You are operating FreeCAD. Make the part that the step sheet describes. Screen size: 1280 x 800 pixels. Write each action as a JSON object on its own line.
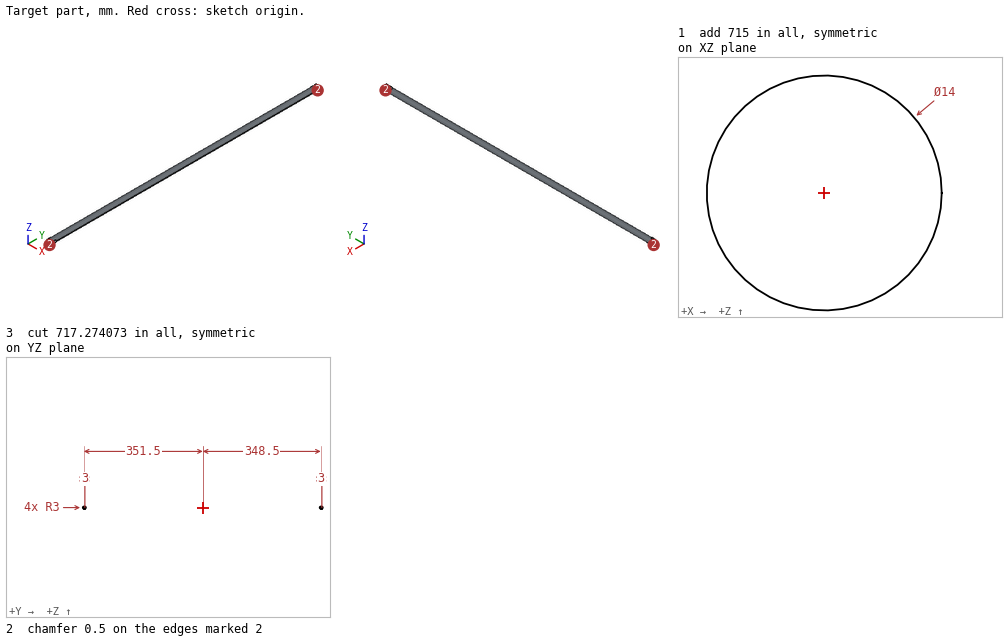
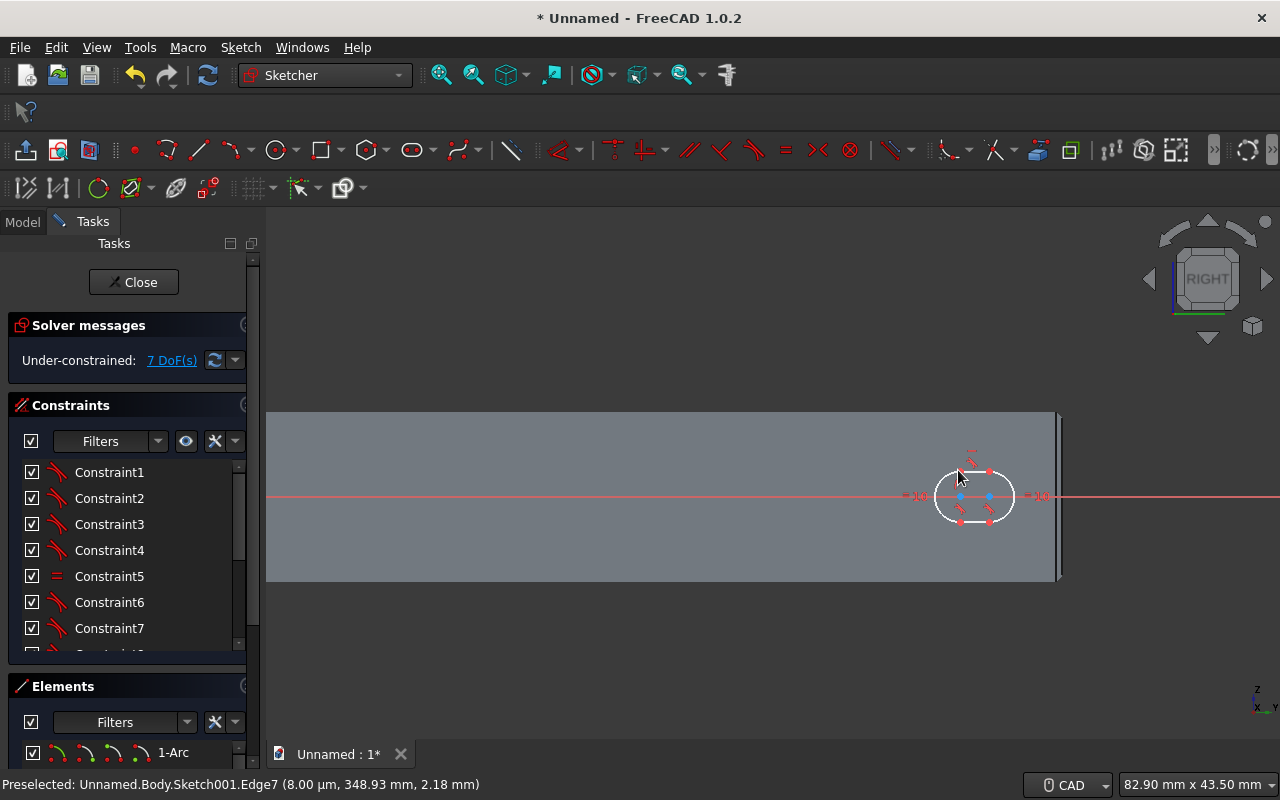
{"action": "scroll", "coordinate": [964, 471], "scroll_direction": "down", "scroll_amount": 14}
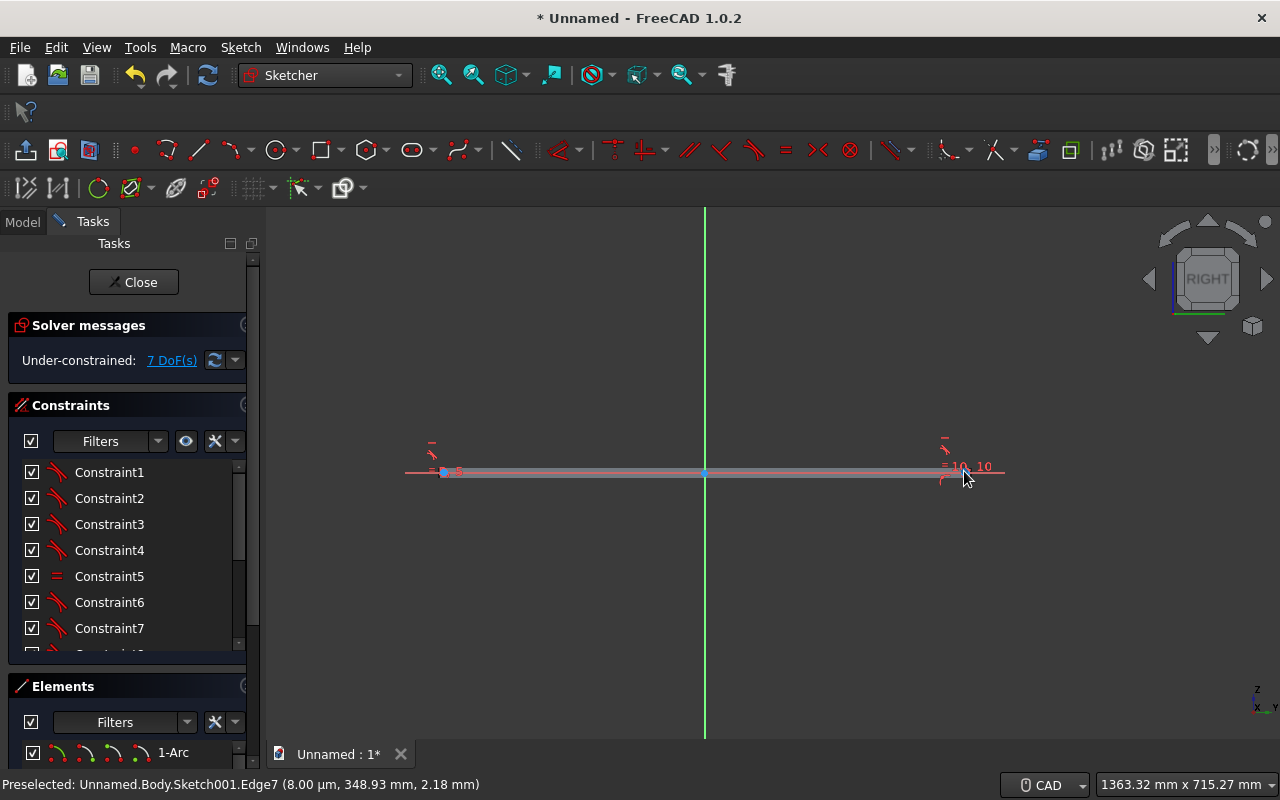
{"action": "scroll", "coordinate": [443, 472], "scroll_direction": "up", "scroll_amount": 14}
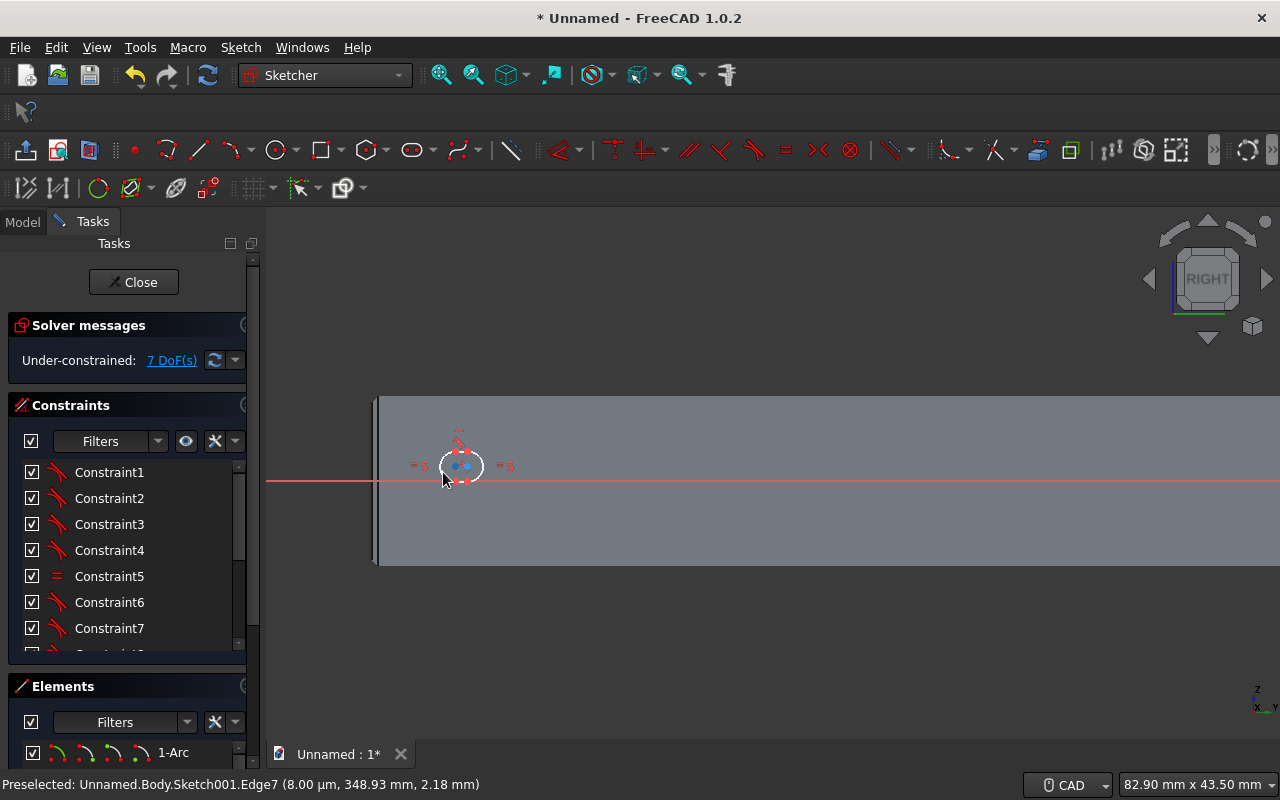
{"action": "left_click", "coordinate": [443, 458]}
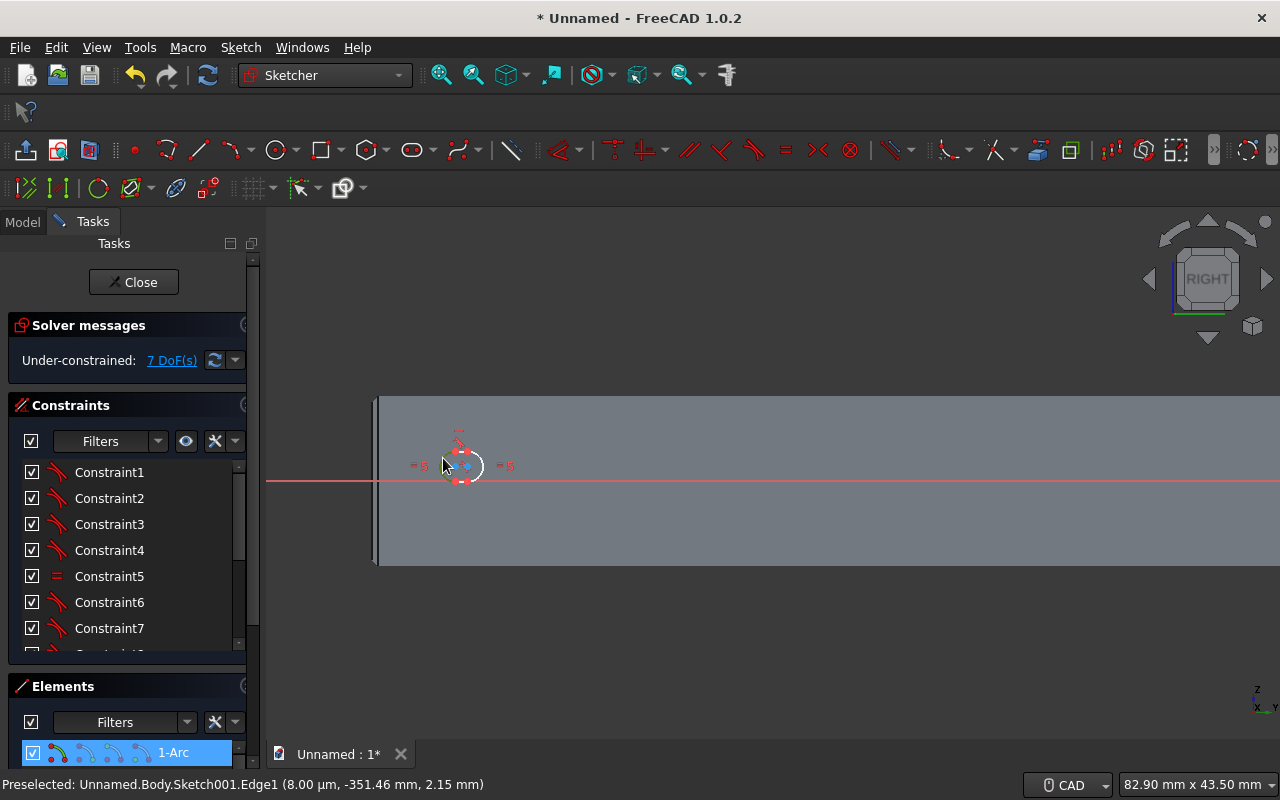
{"action": "scroll", "coordinate": [443, 472], "scroll_direction": "down", "scroll_amount": 14}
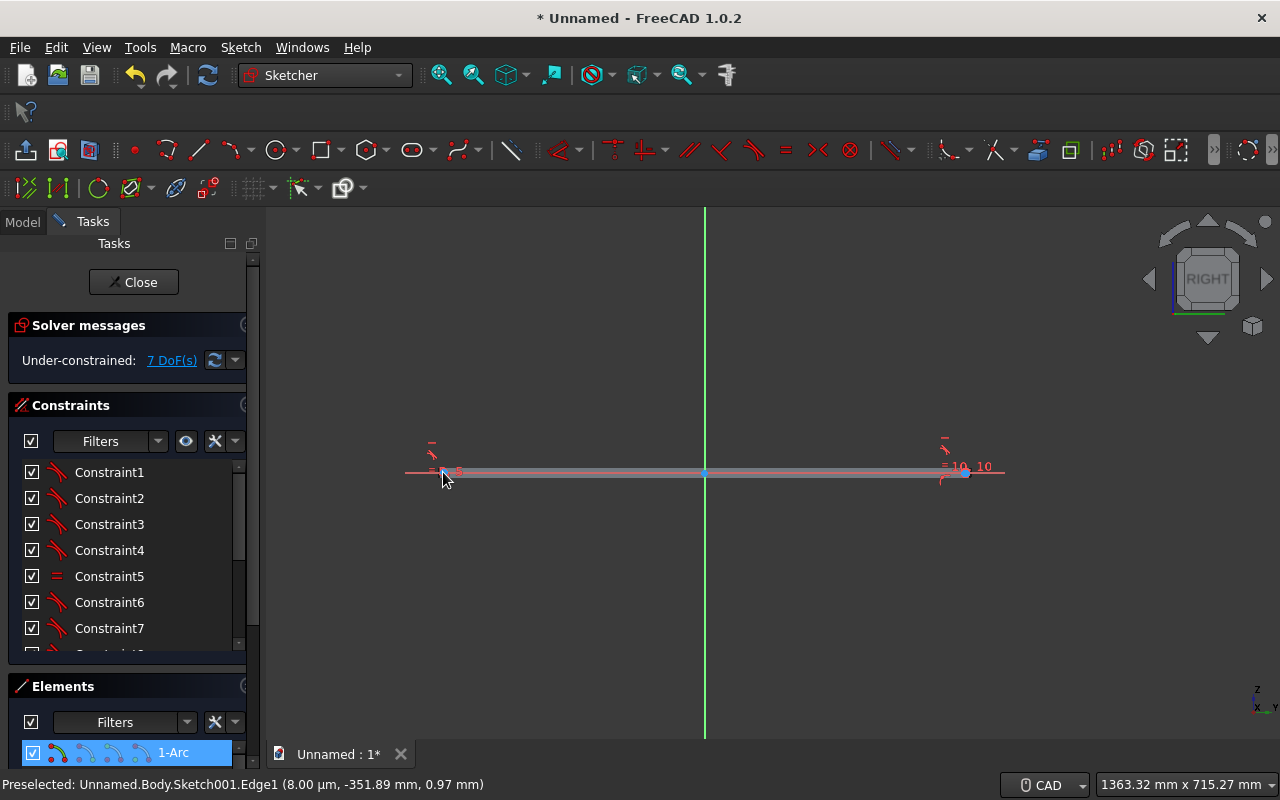
{"action": "scroll", "coordinate": [963, 472], "scroll_direction": "up", "scroll_amount": 14}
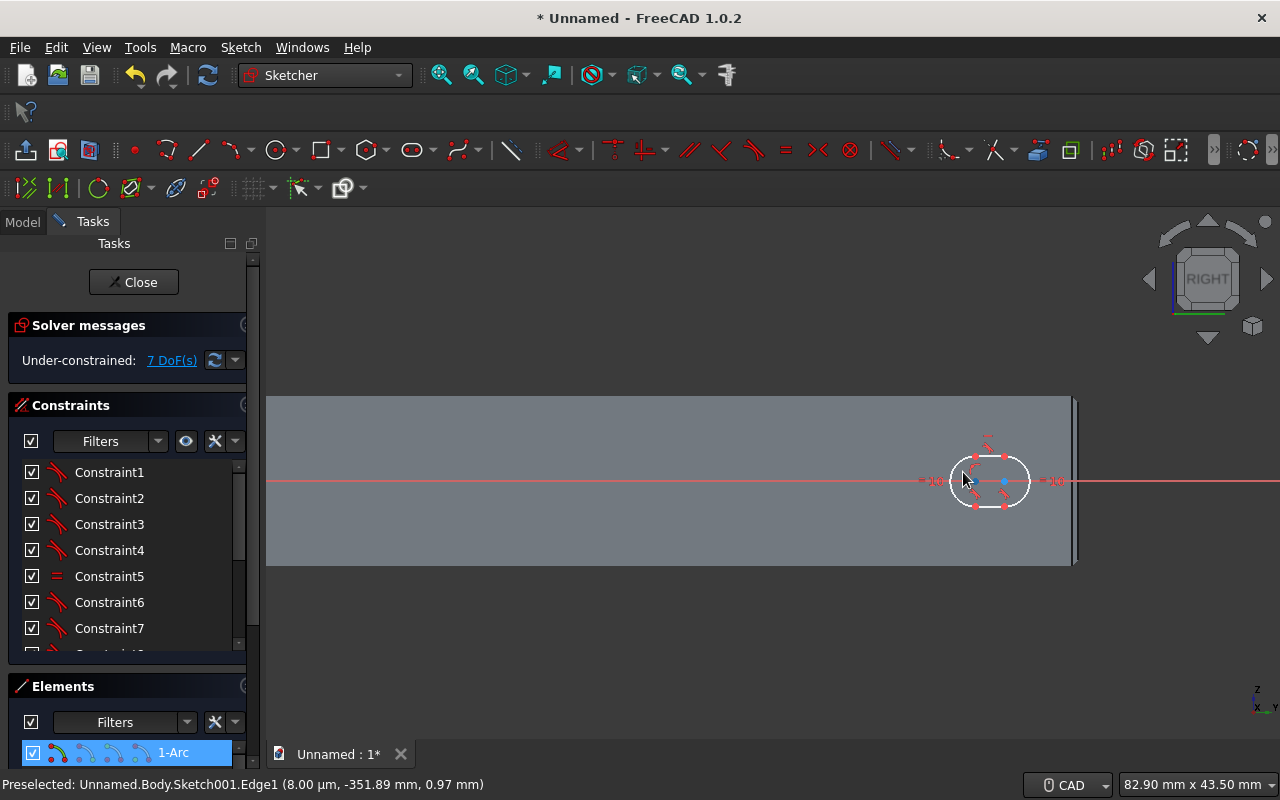
{"action": "left_click", "coordinate": [955, 467]}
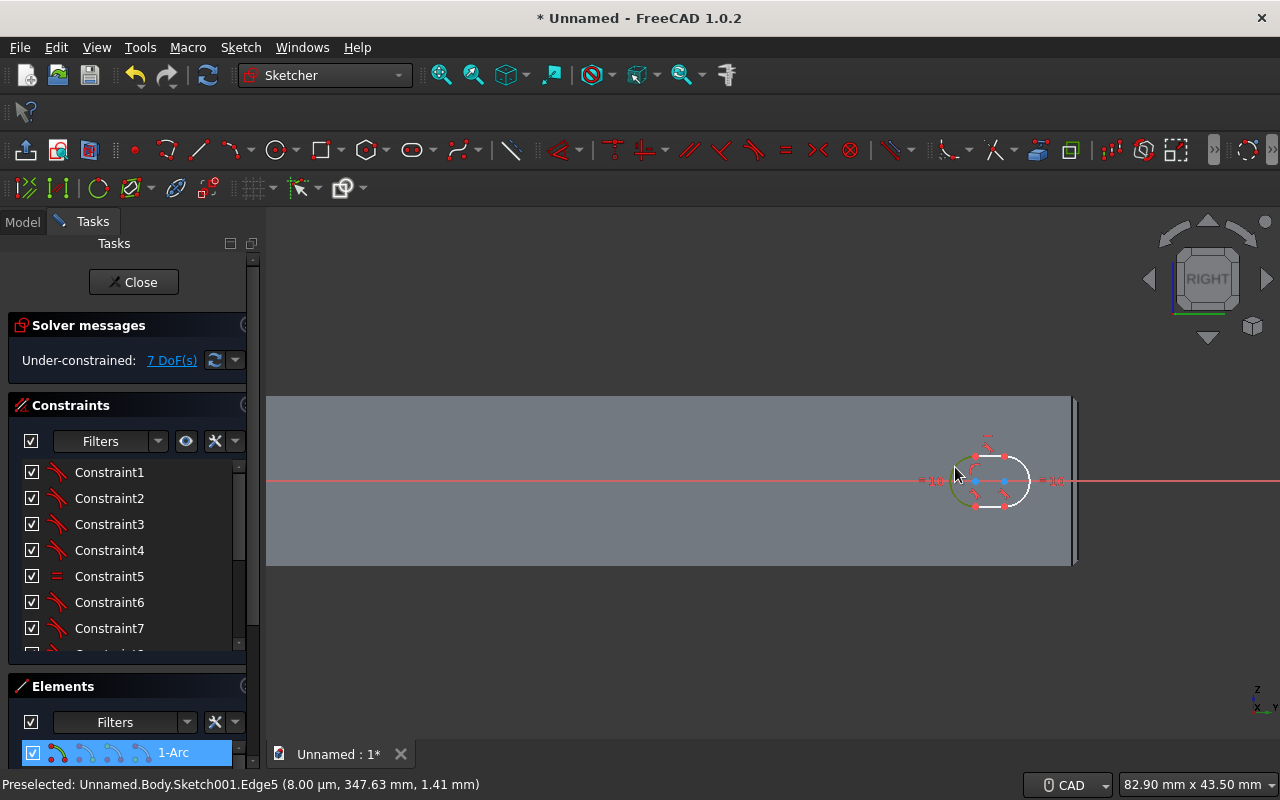
{"action": "left_click", "coordinate": [786, 150]}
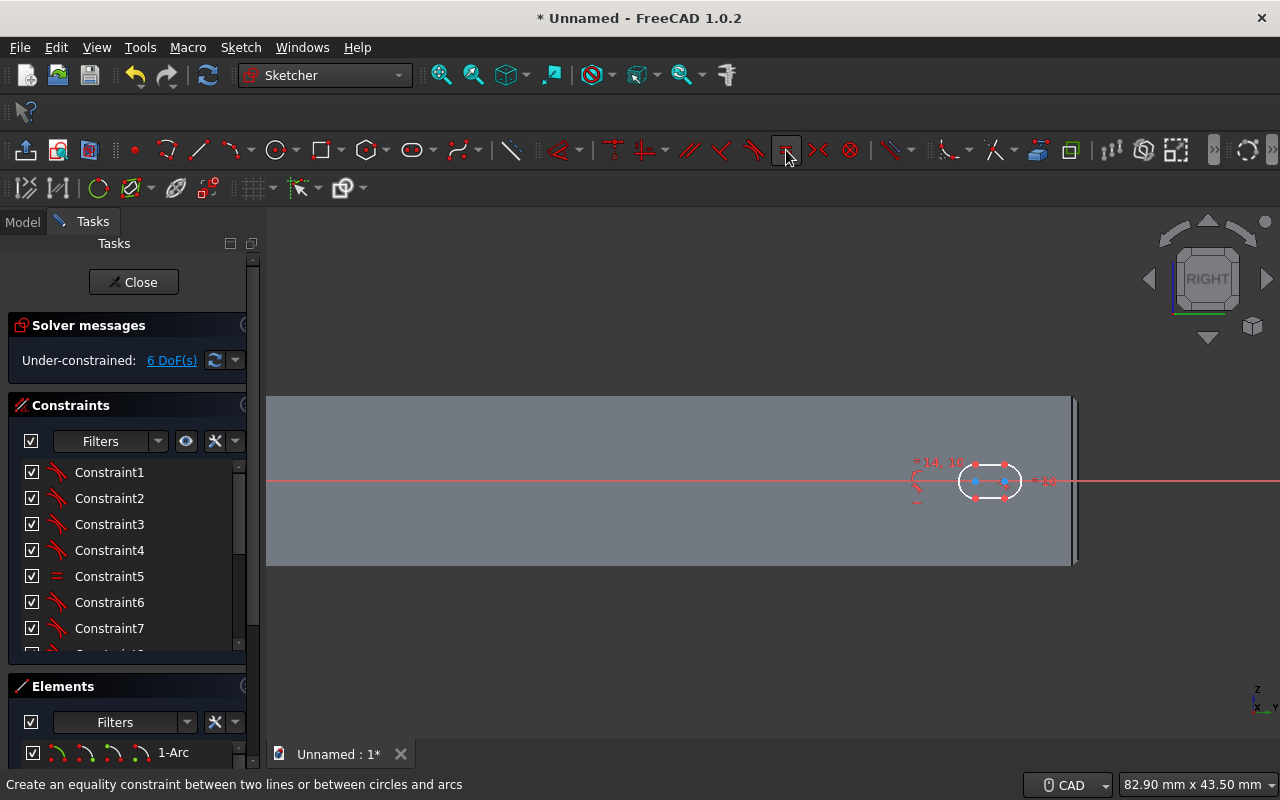
{"action": "scroll", "coordinate": [963, 472], "scroll_direction": "down", "scroll_amount": 14}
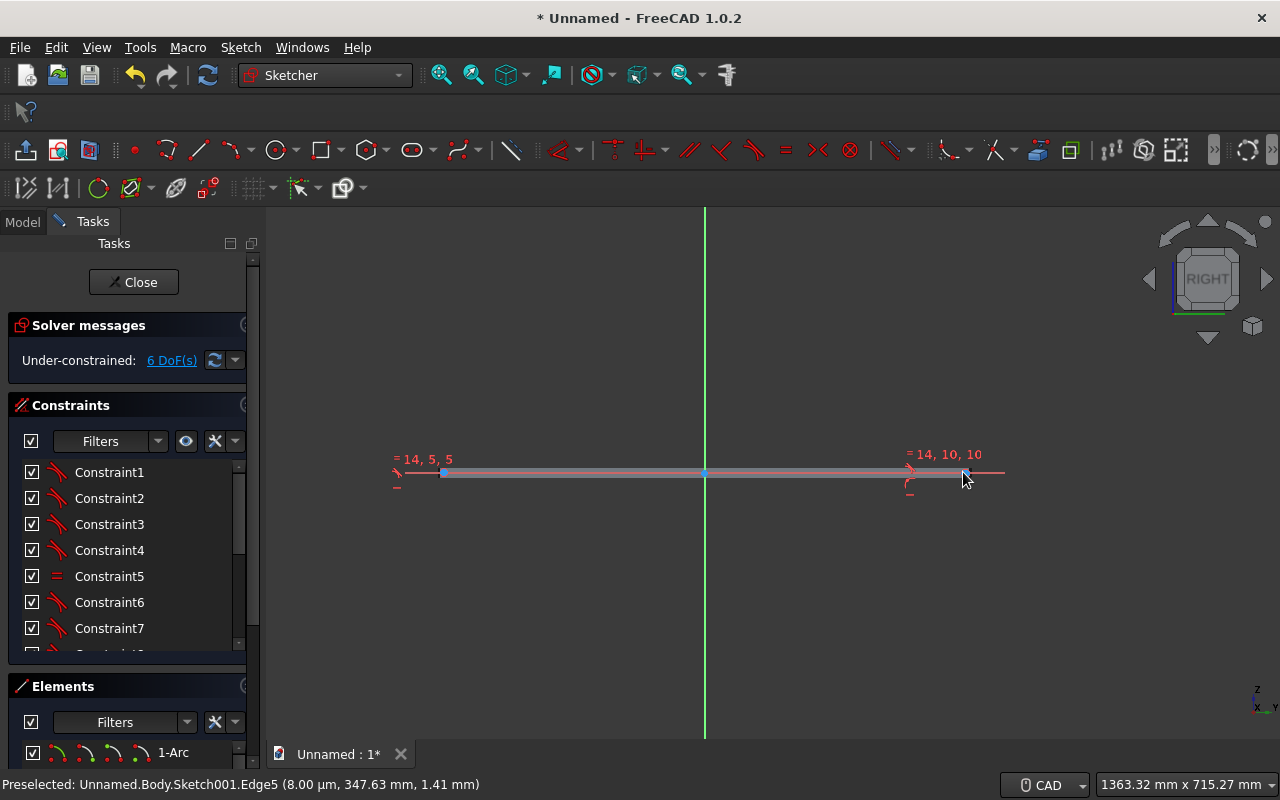
{"action": "scroll", "coordinate": [444, 472], "scroll_direction": "up", "scroll_amount": 14}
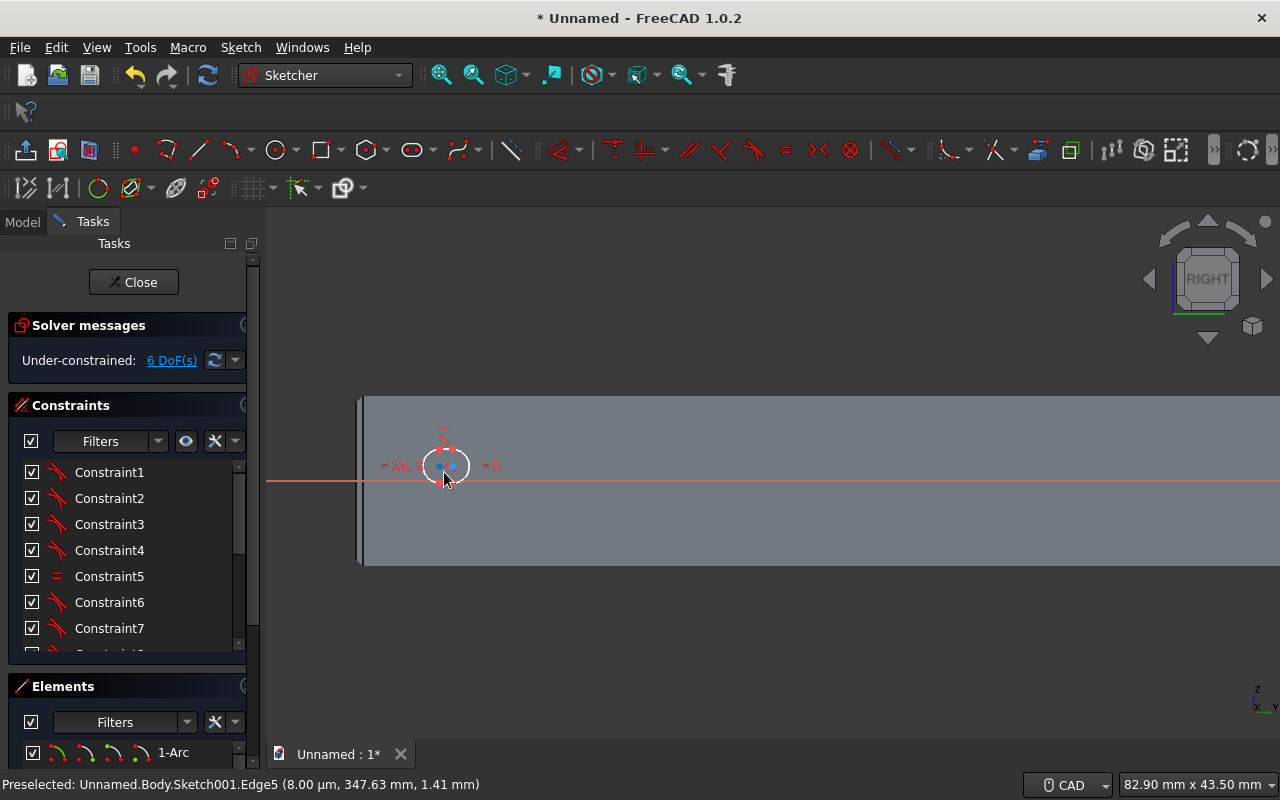
{"action": "left_click", "coordinate": [440, 466]}